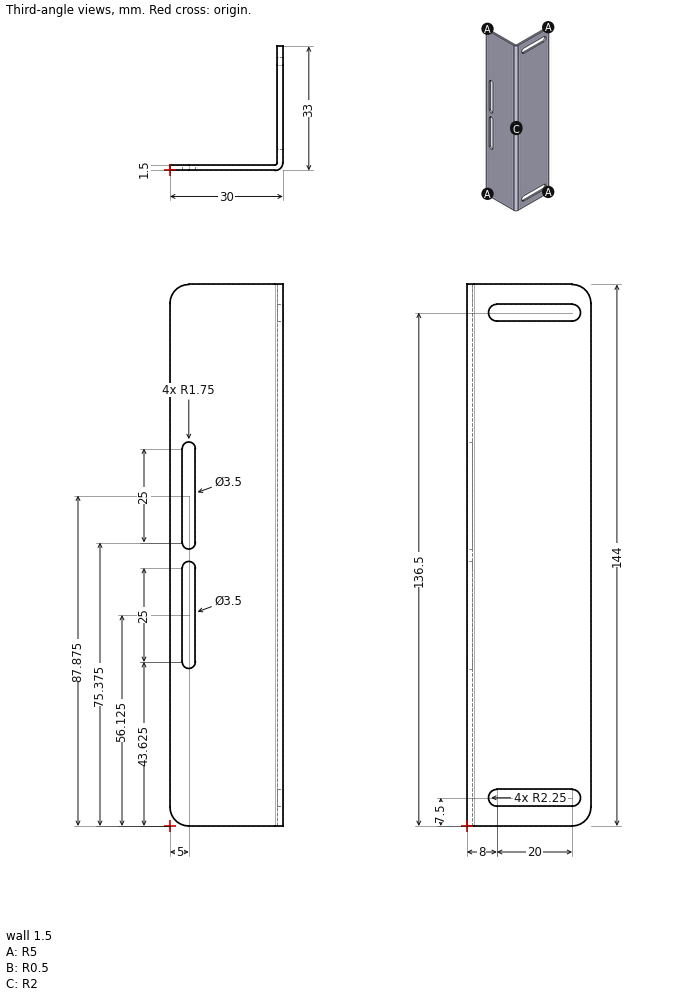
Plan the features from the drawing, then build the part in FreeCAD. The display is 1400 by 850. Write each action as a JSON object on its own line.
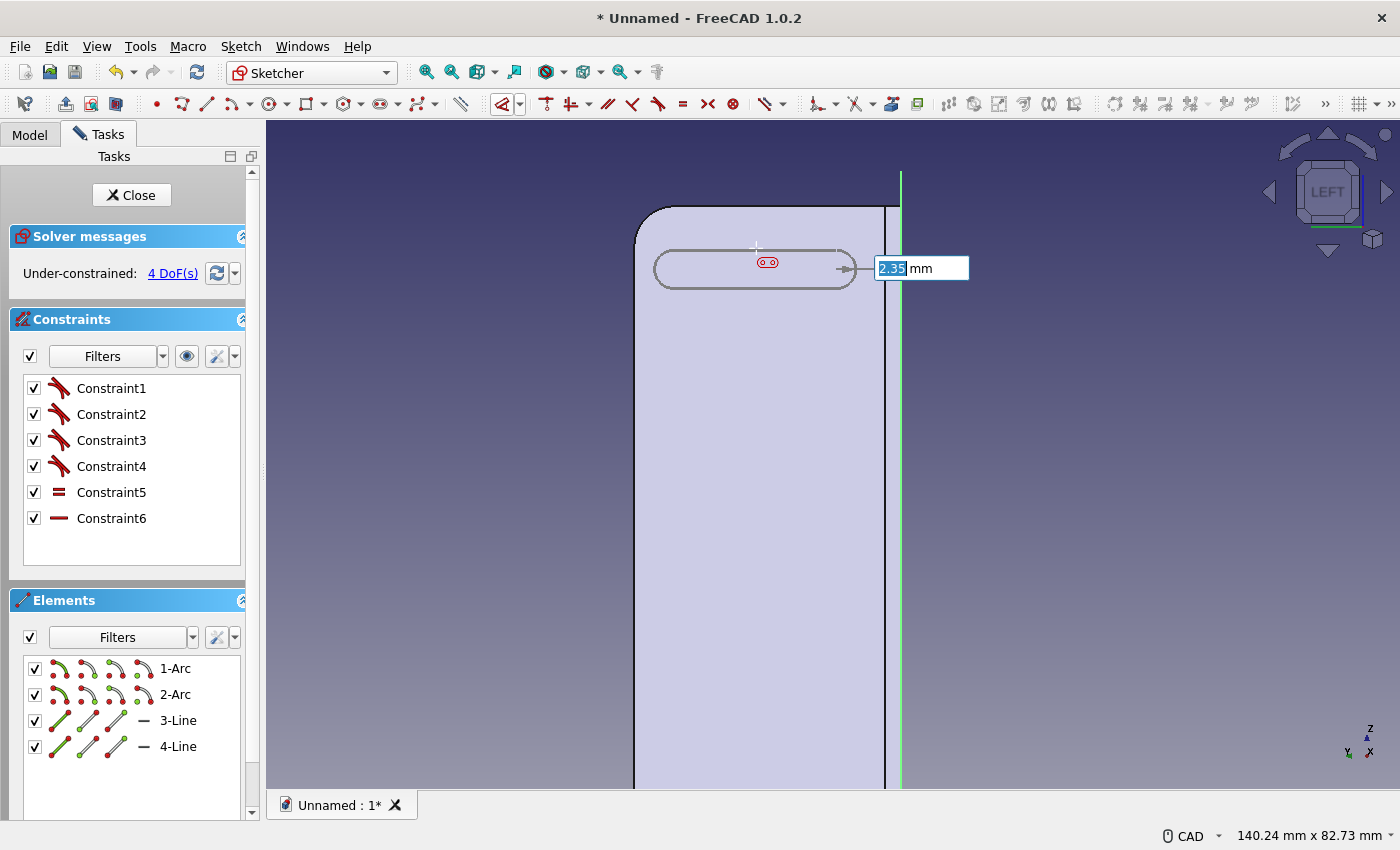
{"action": "left_click", "coordinate": [756, 249]}
{"action": "key", "text": "Escape"}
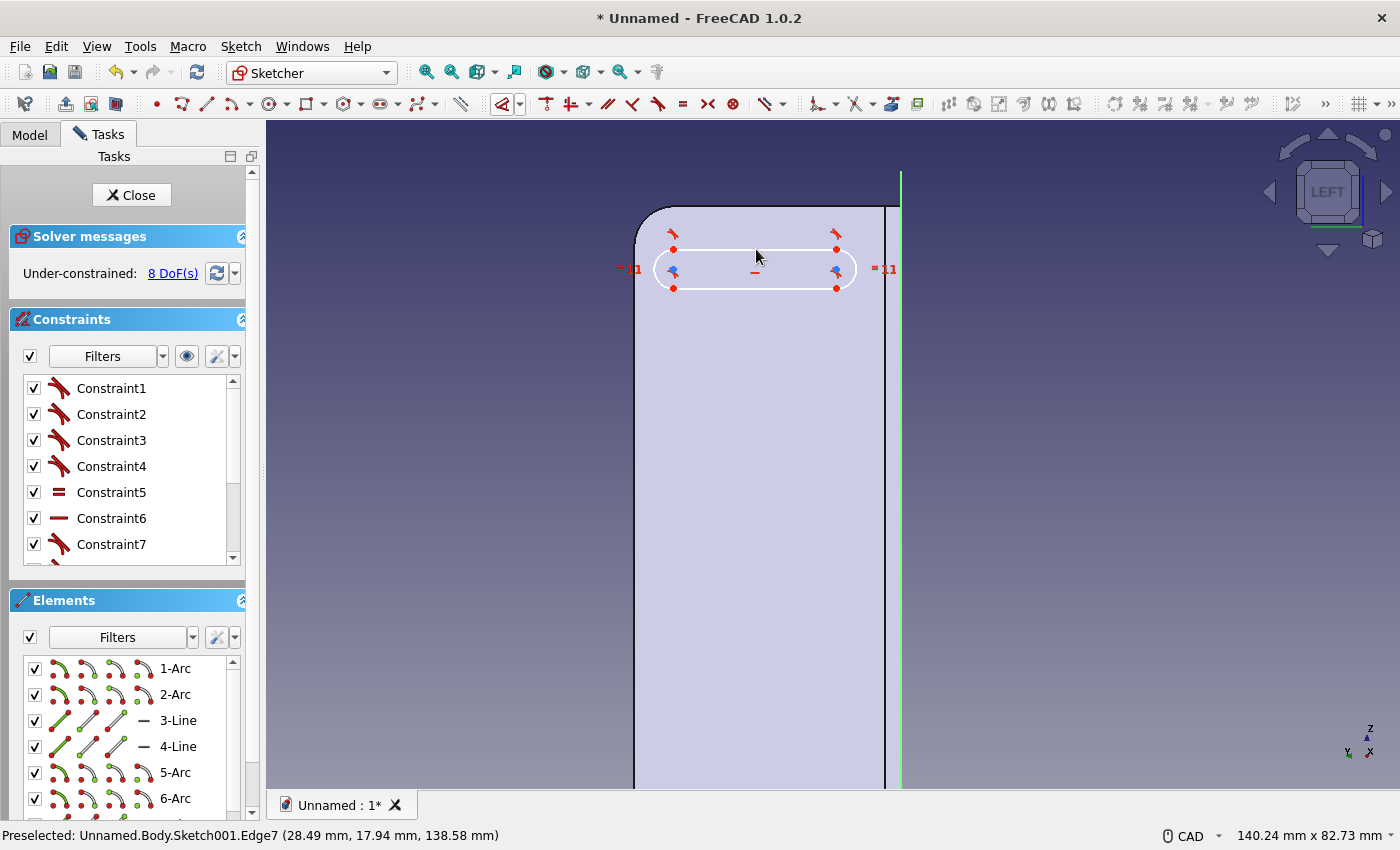
{"action": "scroll", "coordinate": [756, 248], "scroll_direction": "down", "scroll_amount": 5}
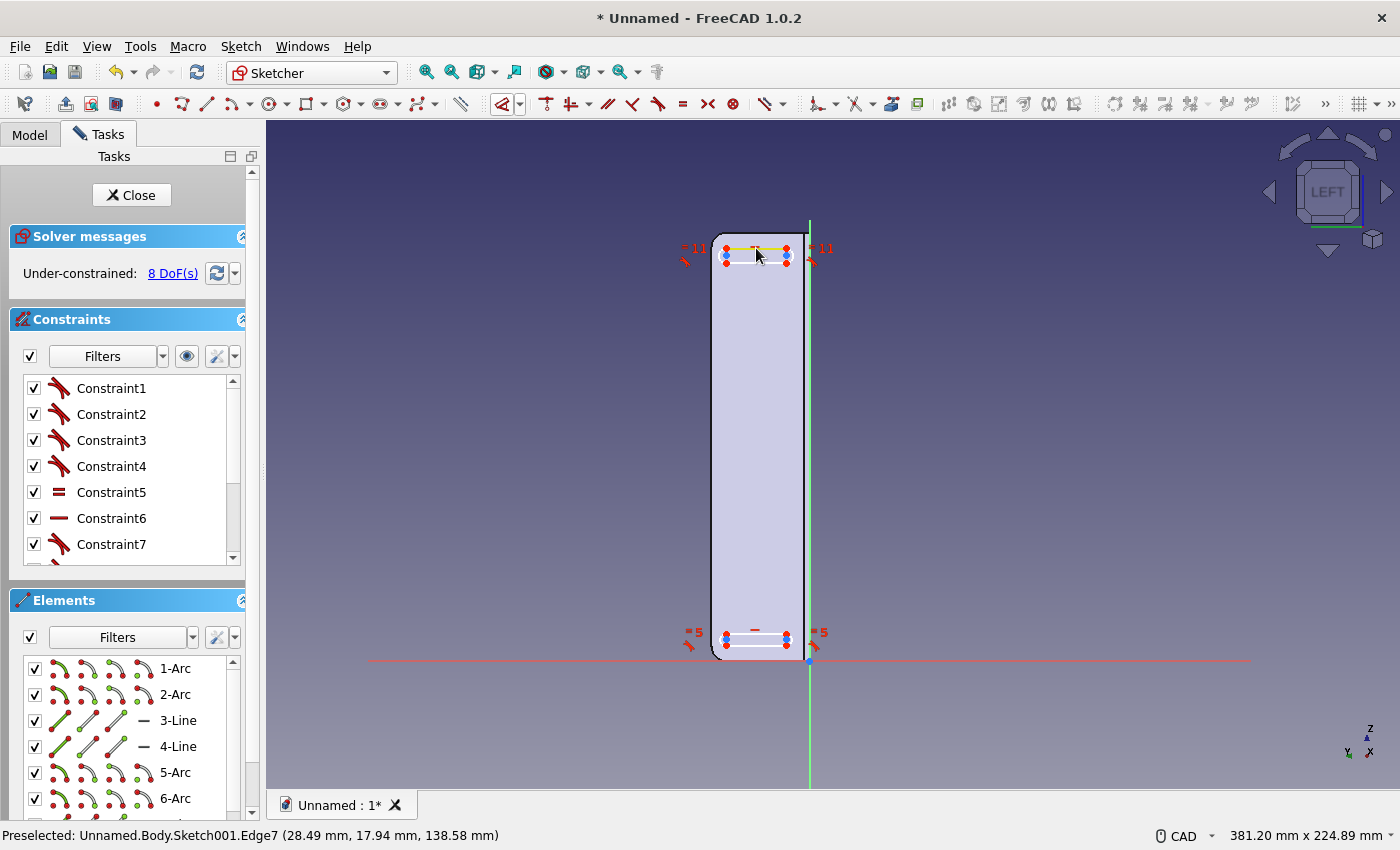
{"action": "scroll", "coordinate": [721, 637], "scroll_direction": "up", "scroll_amount": 5}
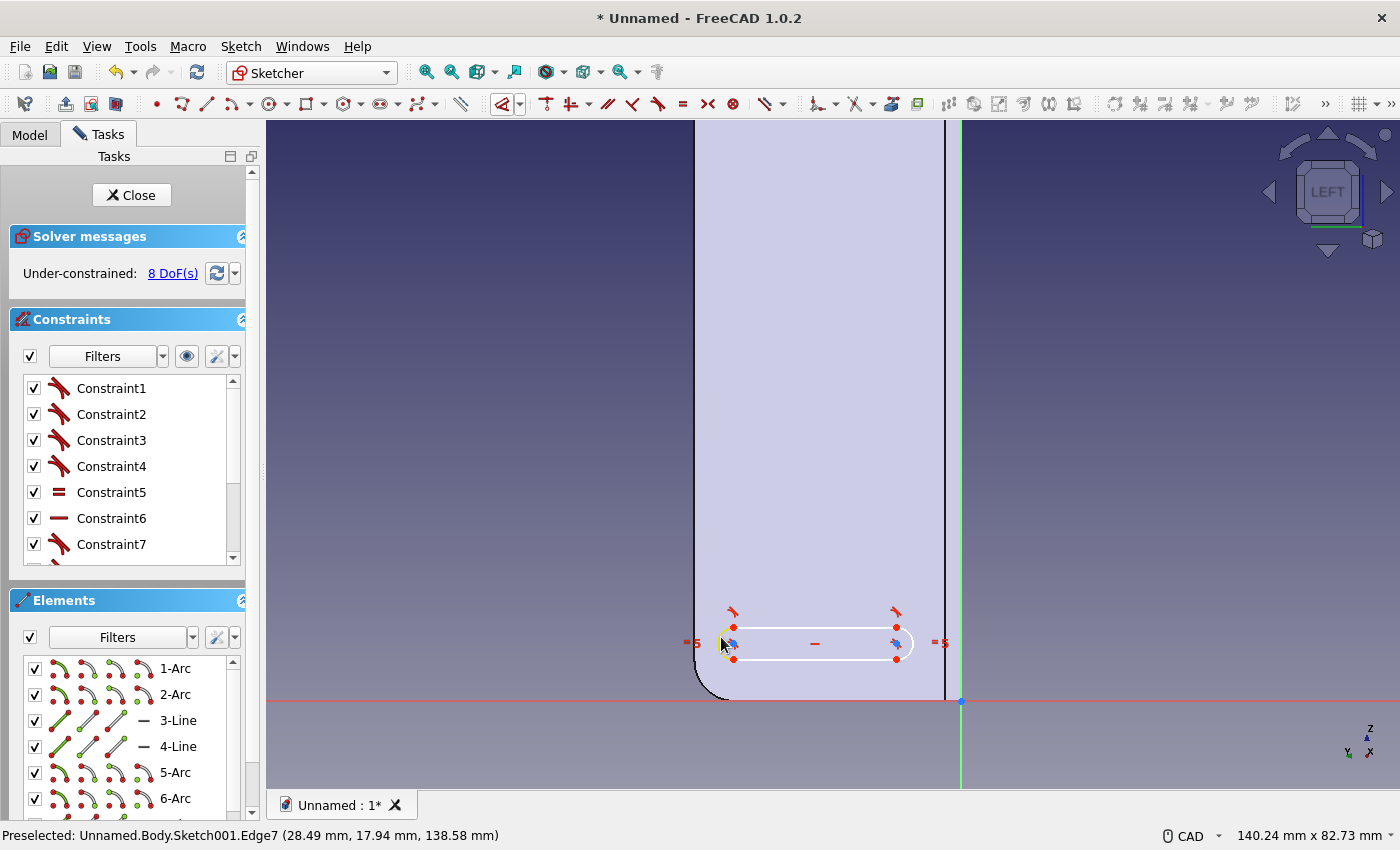
{"action": "left_click", "coordinate": [721, 634]}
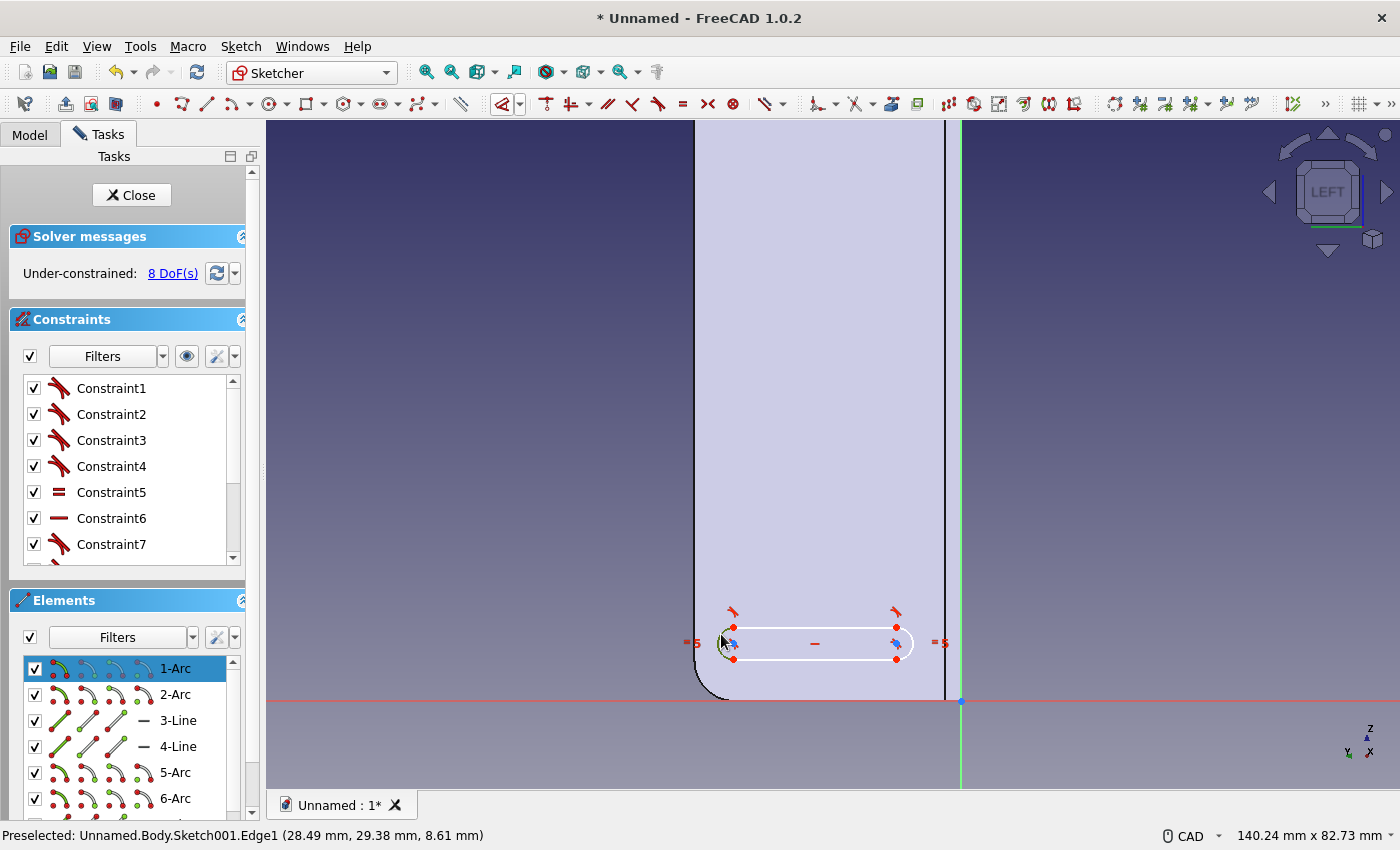
{"action": "scroll", "coordinate": [721, 637], "scroll_direction": "down", "scroll_amount": 5}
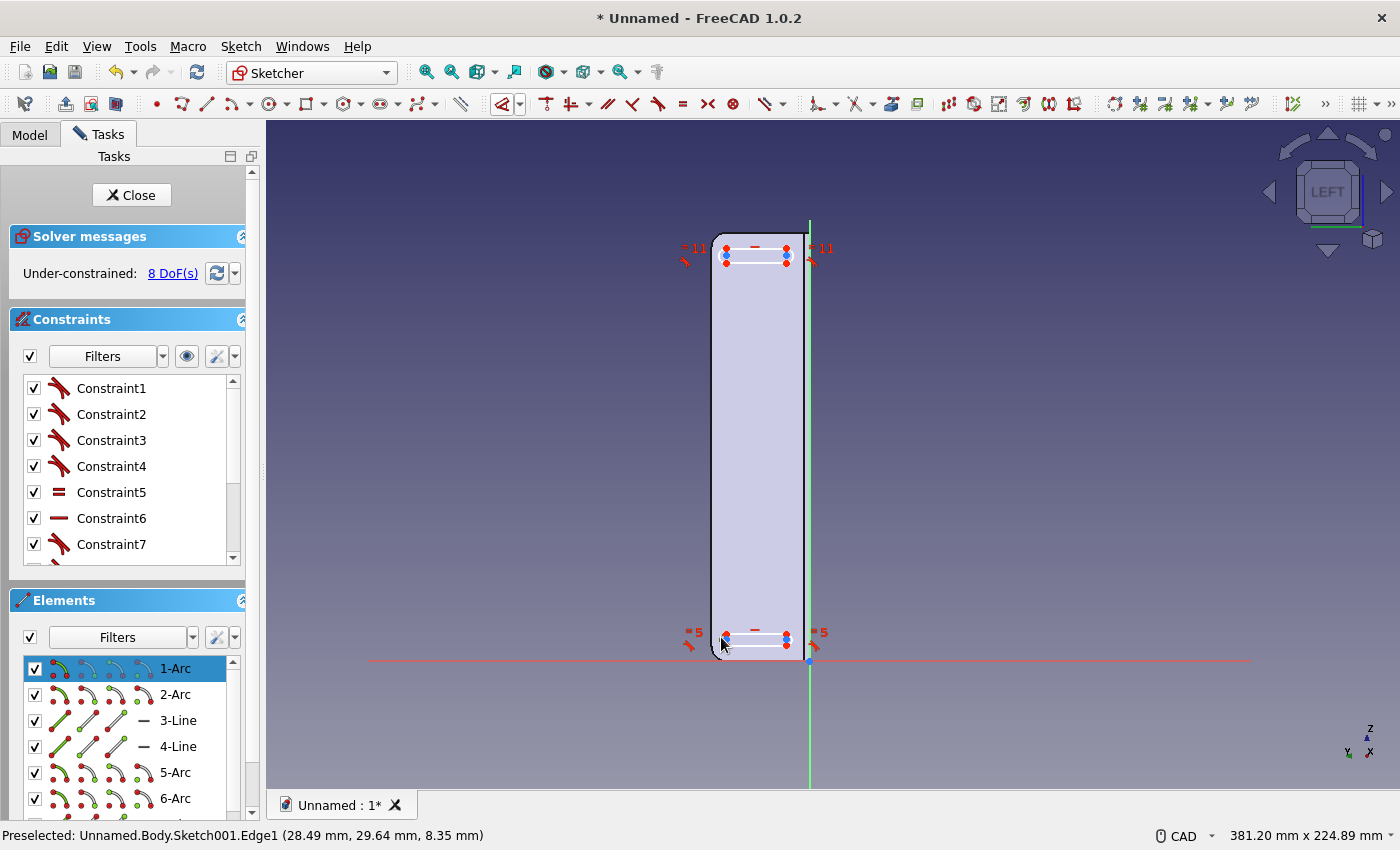
{"action": "scroll", "coordinate": [720, 252], "scroll_direction": "up", "scroll_amount": 4}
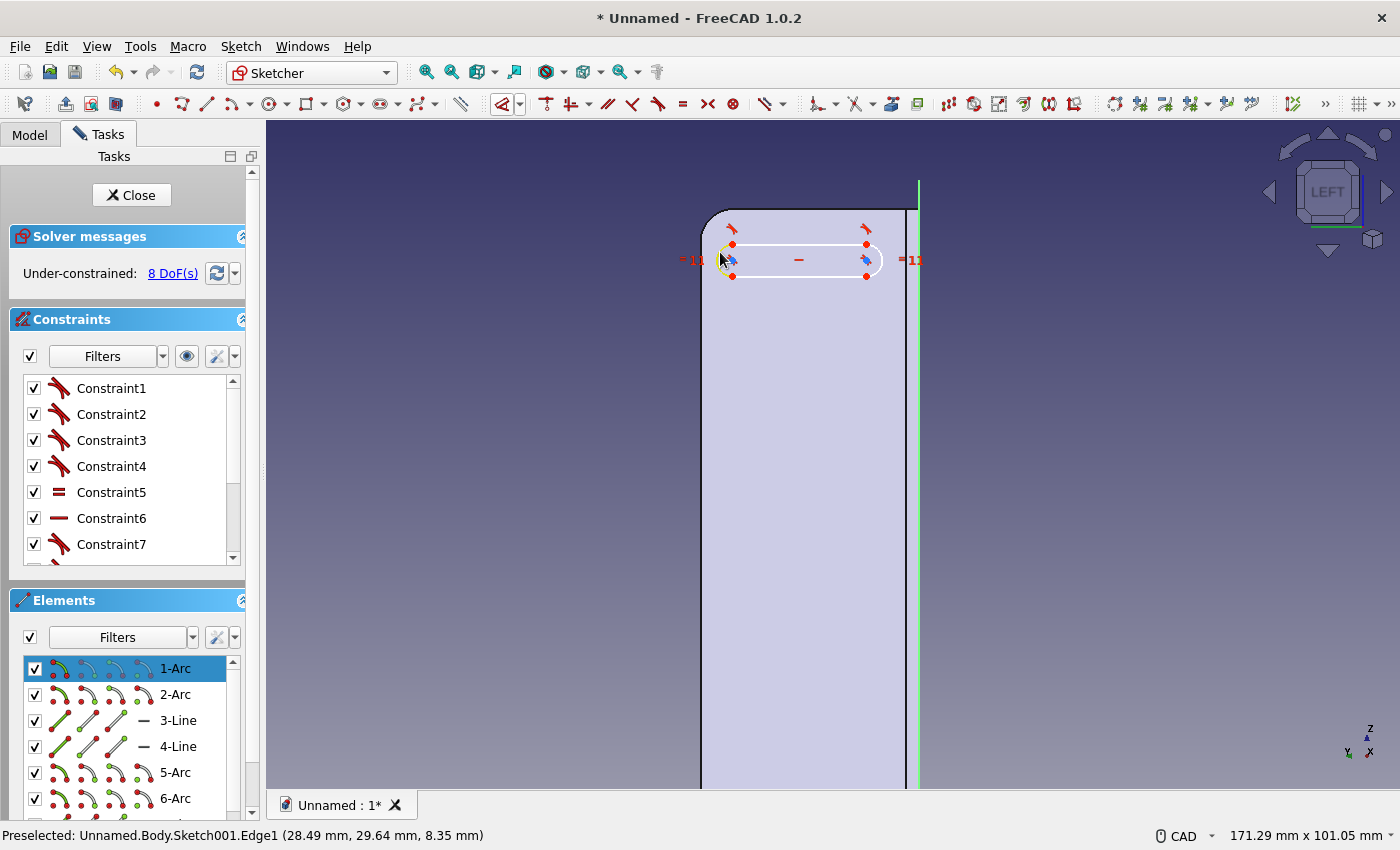
{"action": "left_click", "coordinate": [720, 251]}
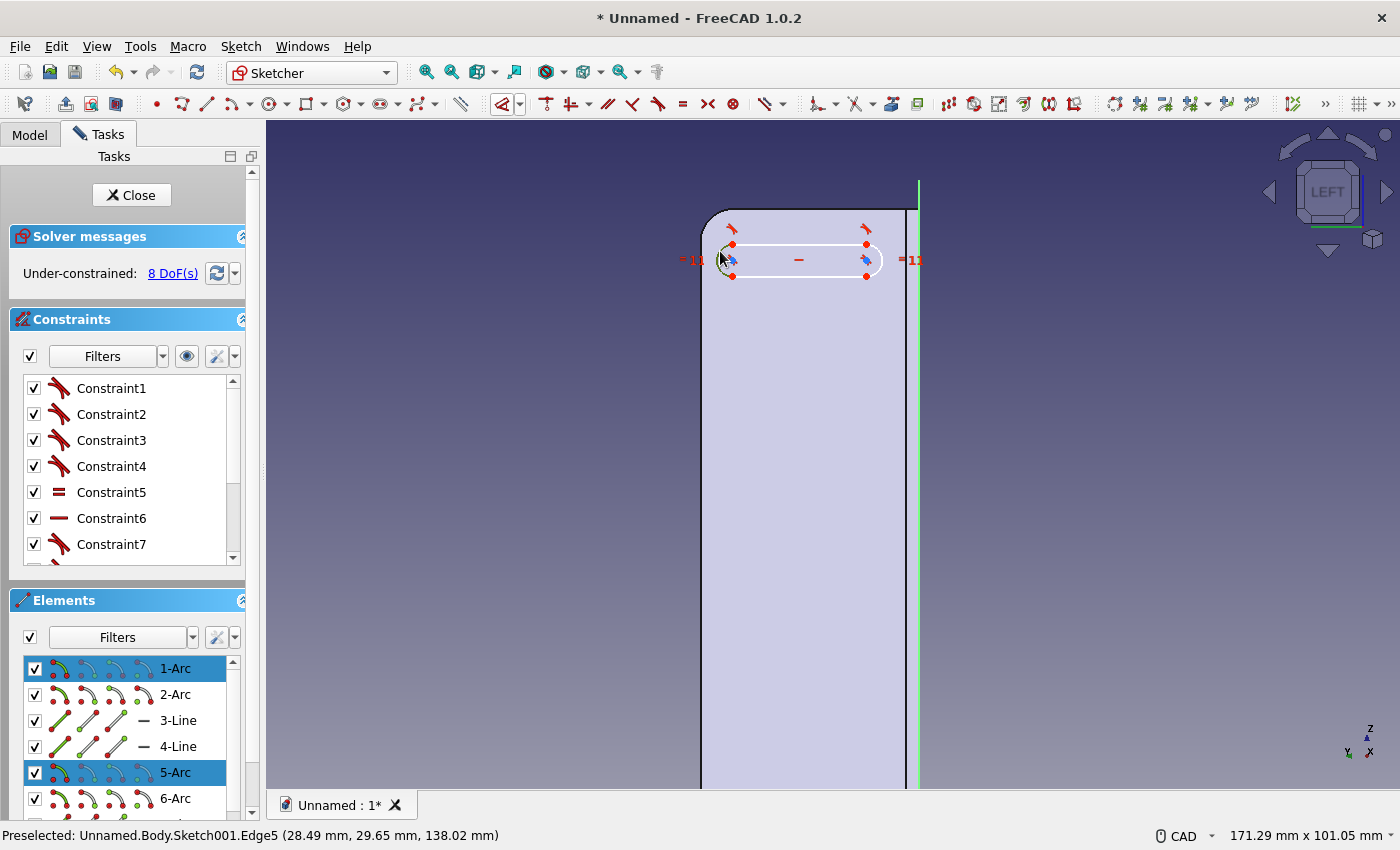
{"action": "left_click", "coordinate": [683, 104]}